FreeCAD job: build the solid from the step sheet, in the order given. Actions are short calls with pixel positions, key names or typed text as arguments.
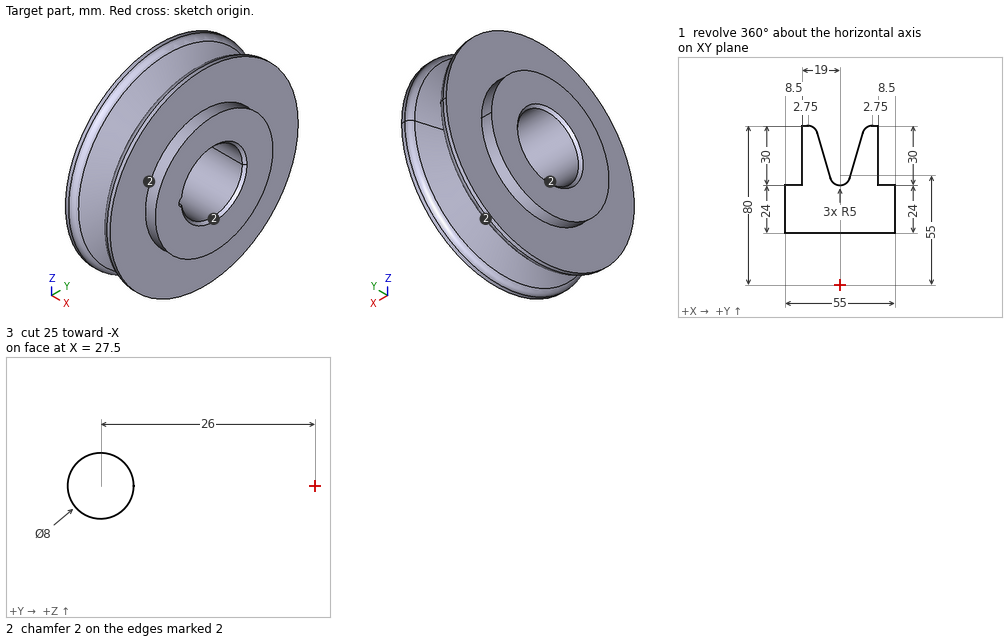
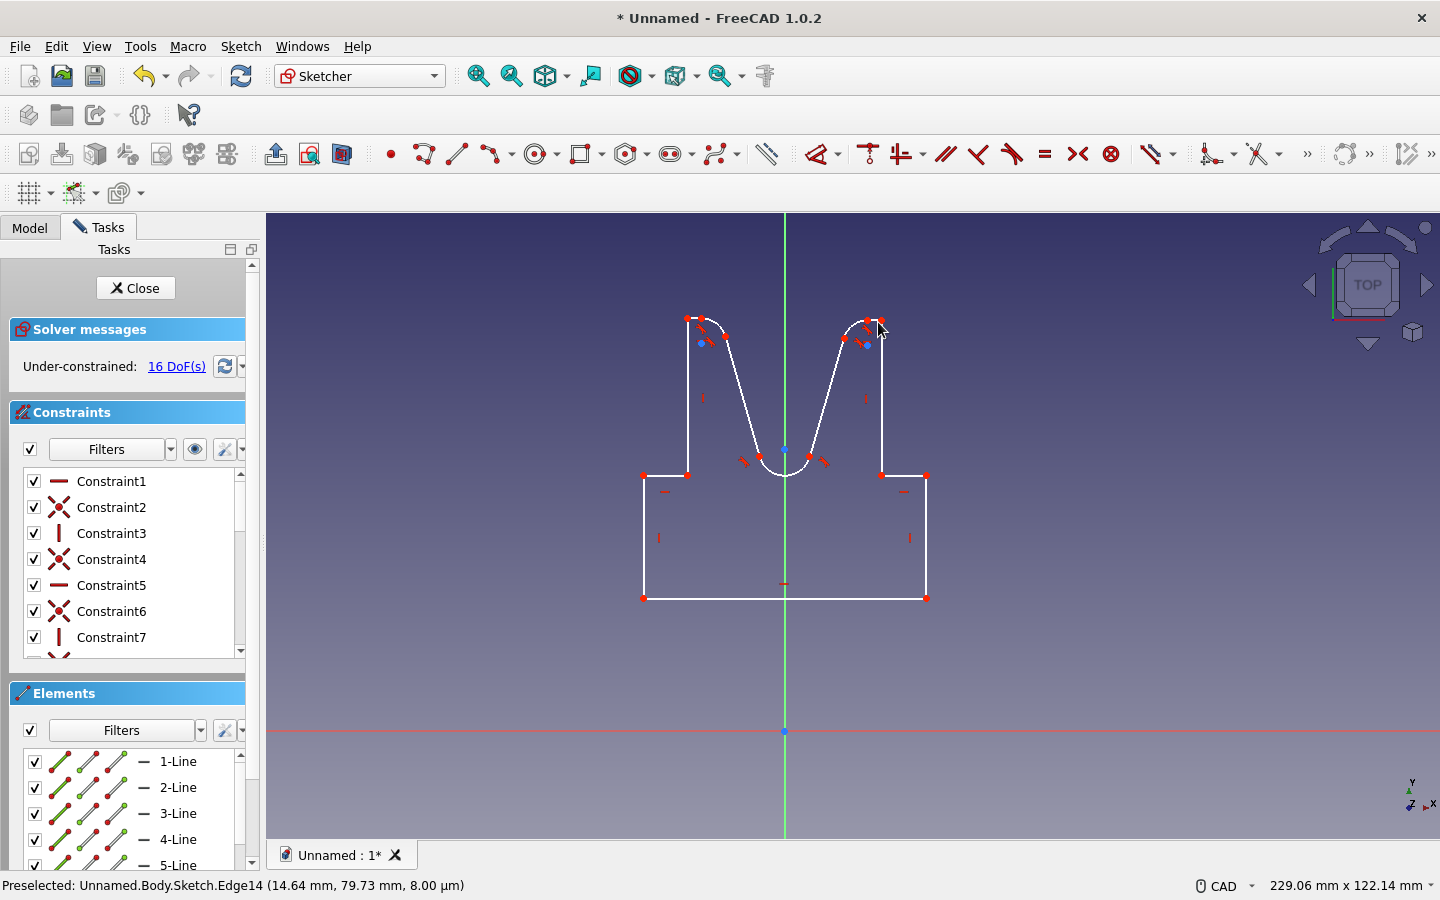
click(767, 468)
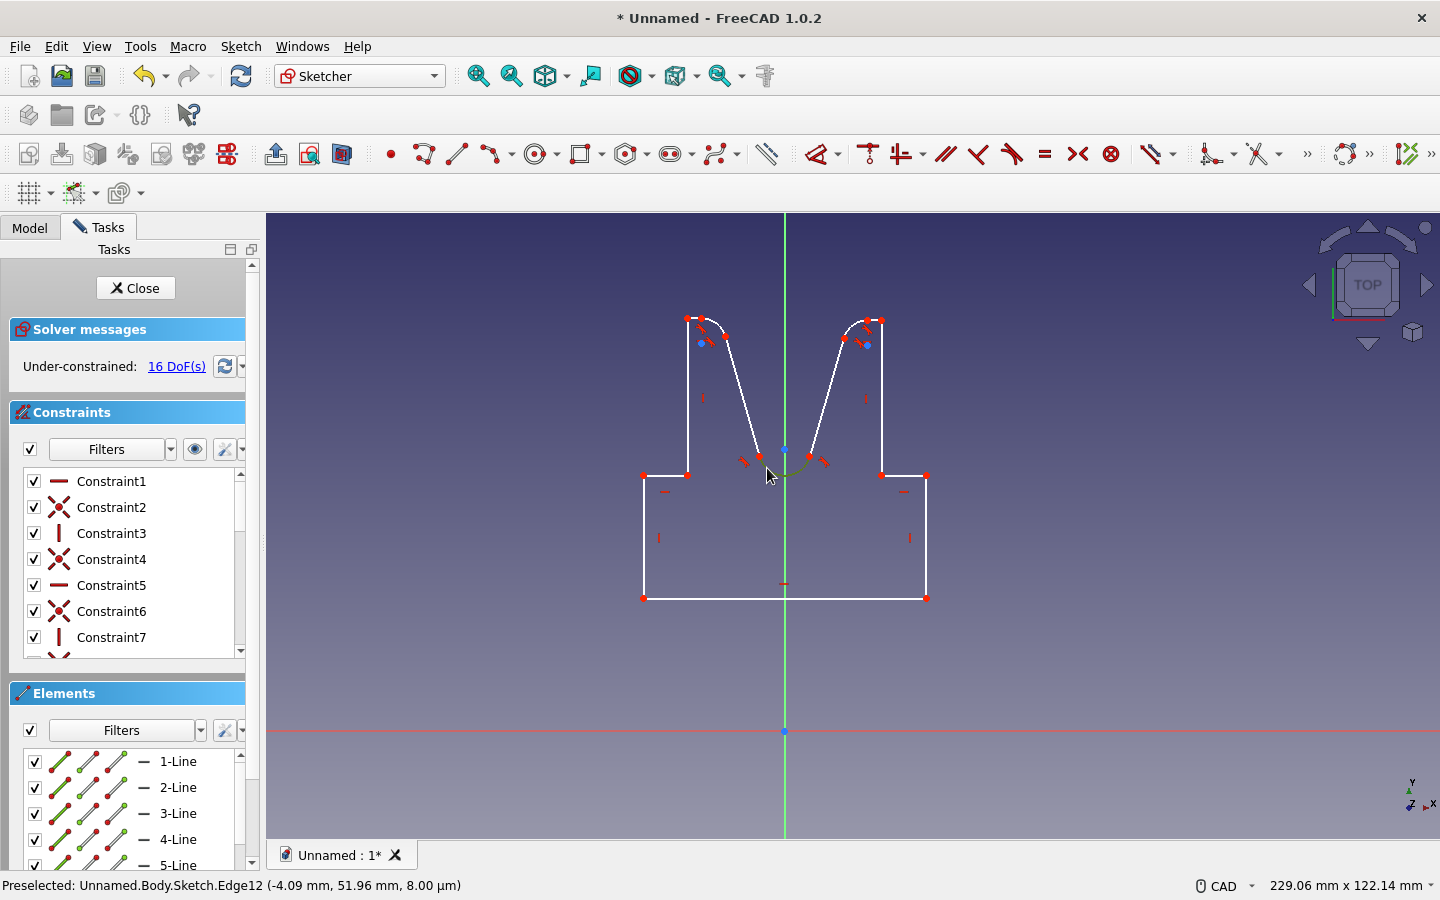
scroll(721, 328, up, 2)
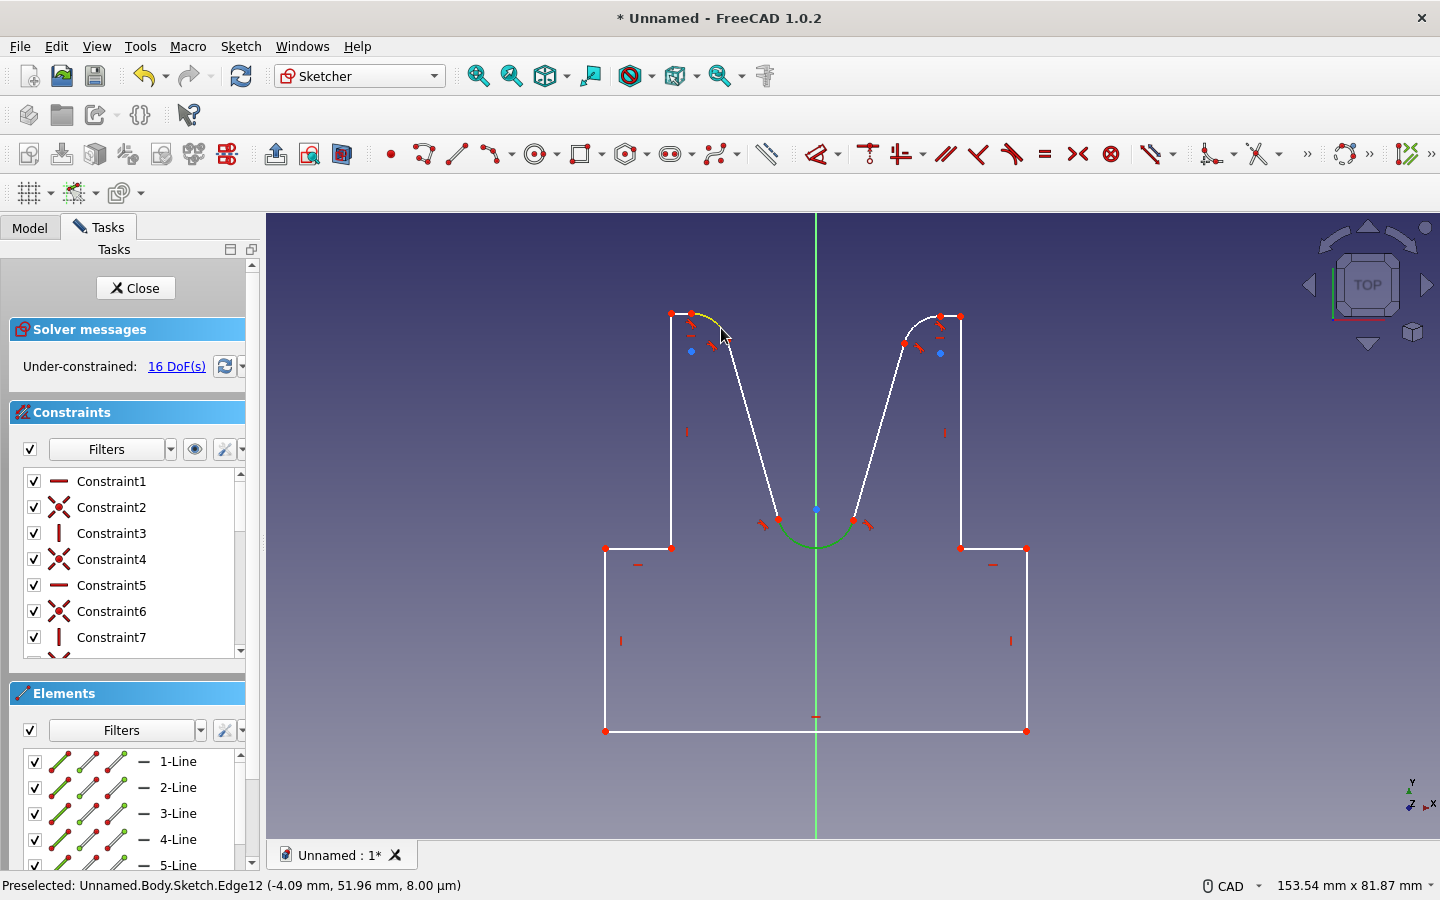
click(721, 328)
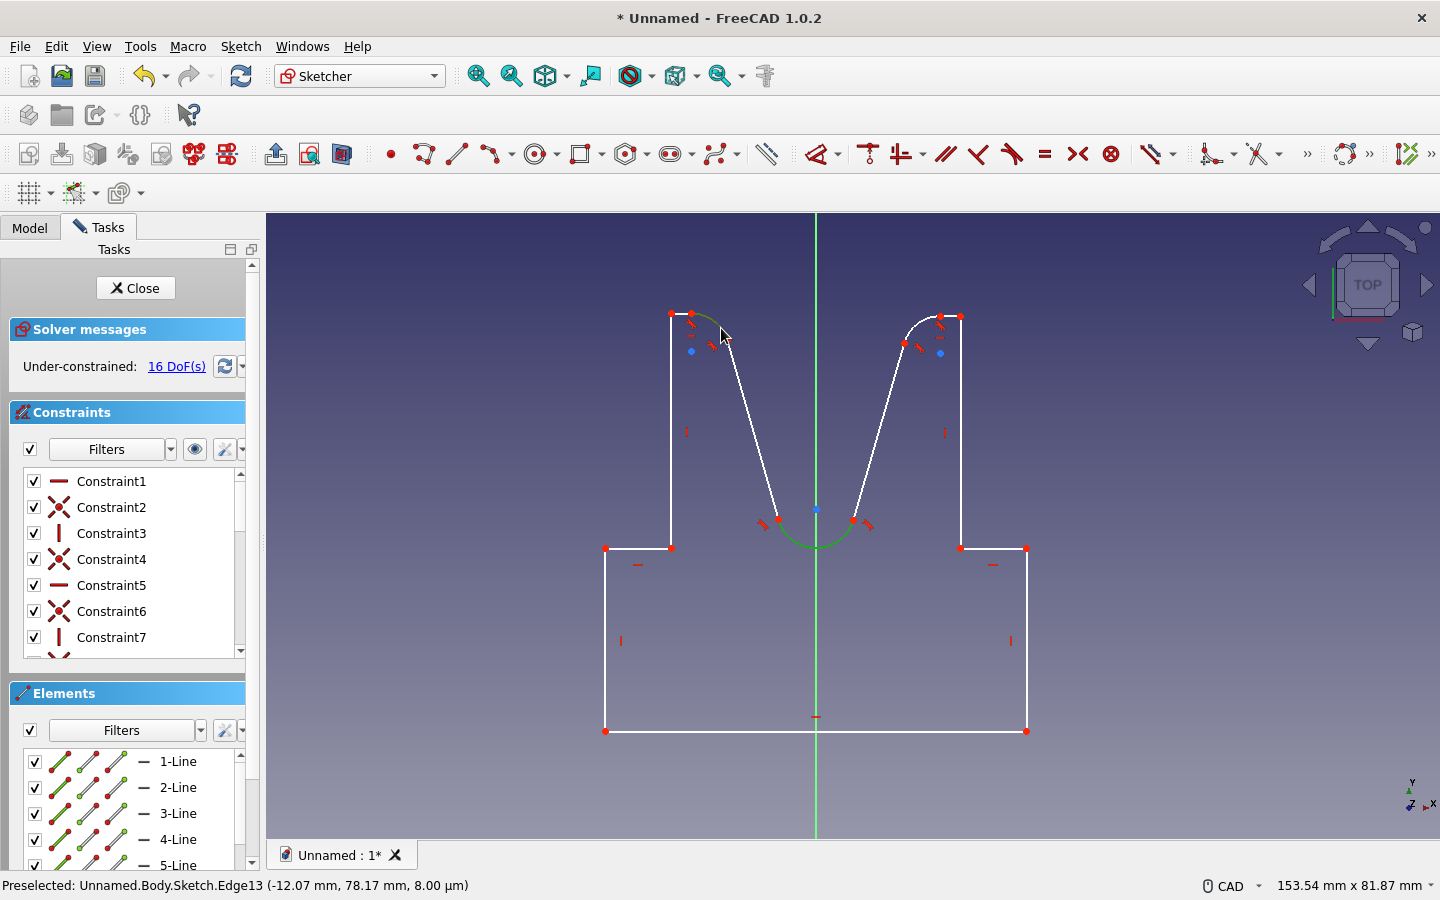
click(926, 319)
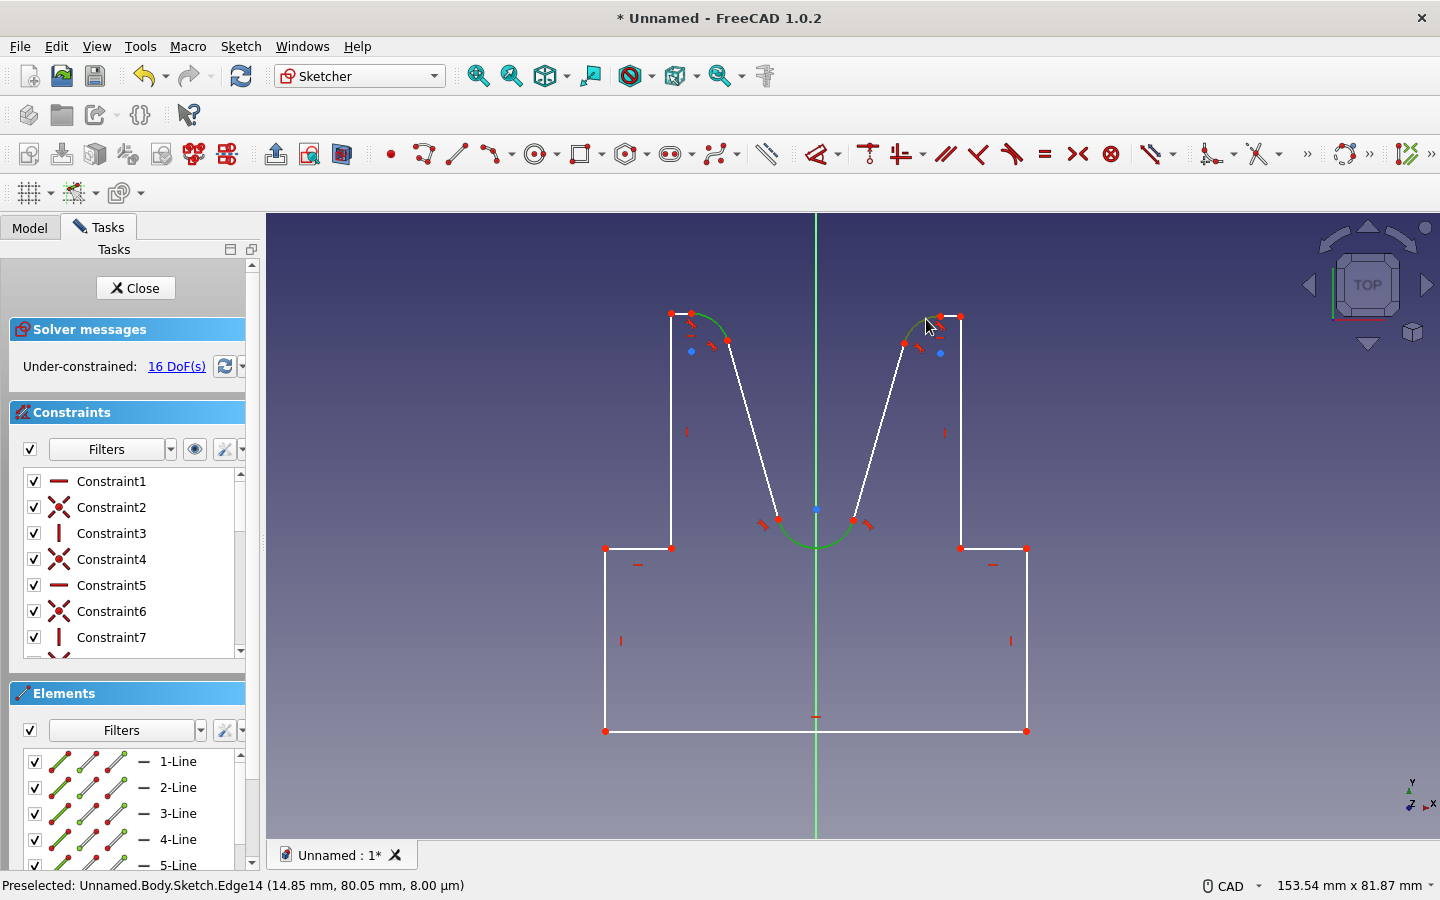
key(e)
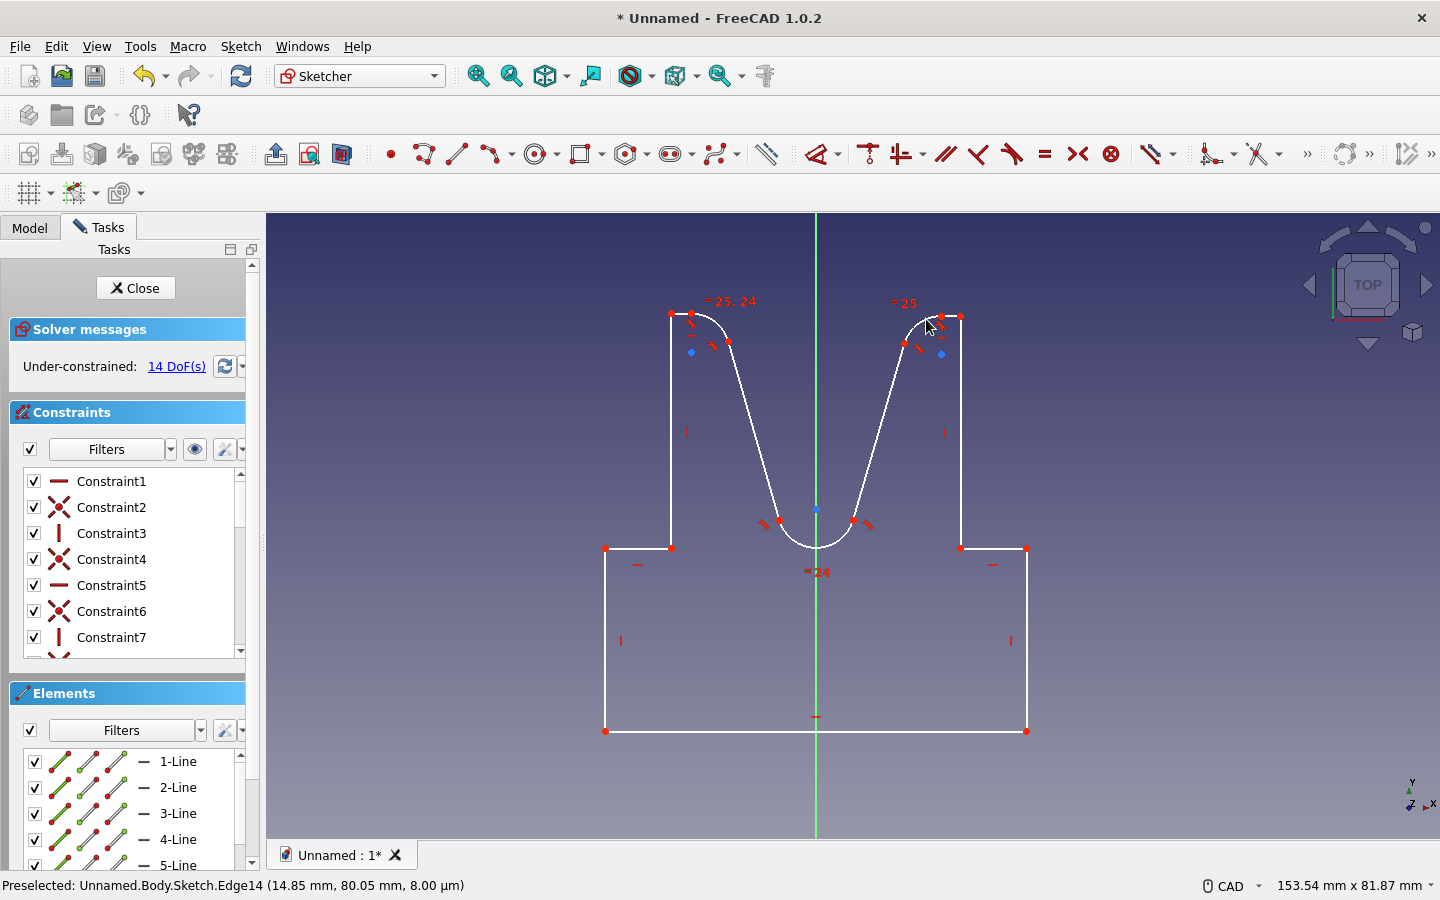
click(816, 509)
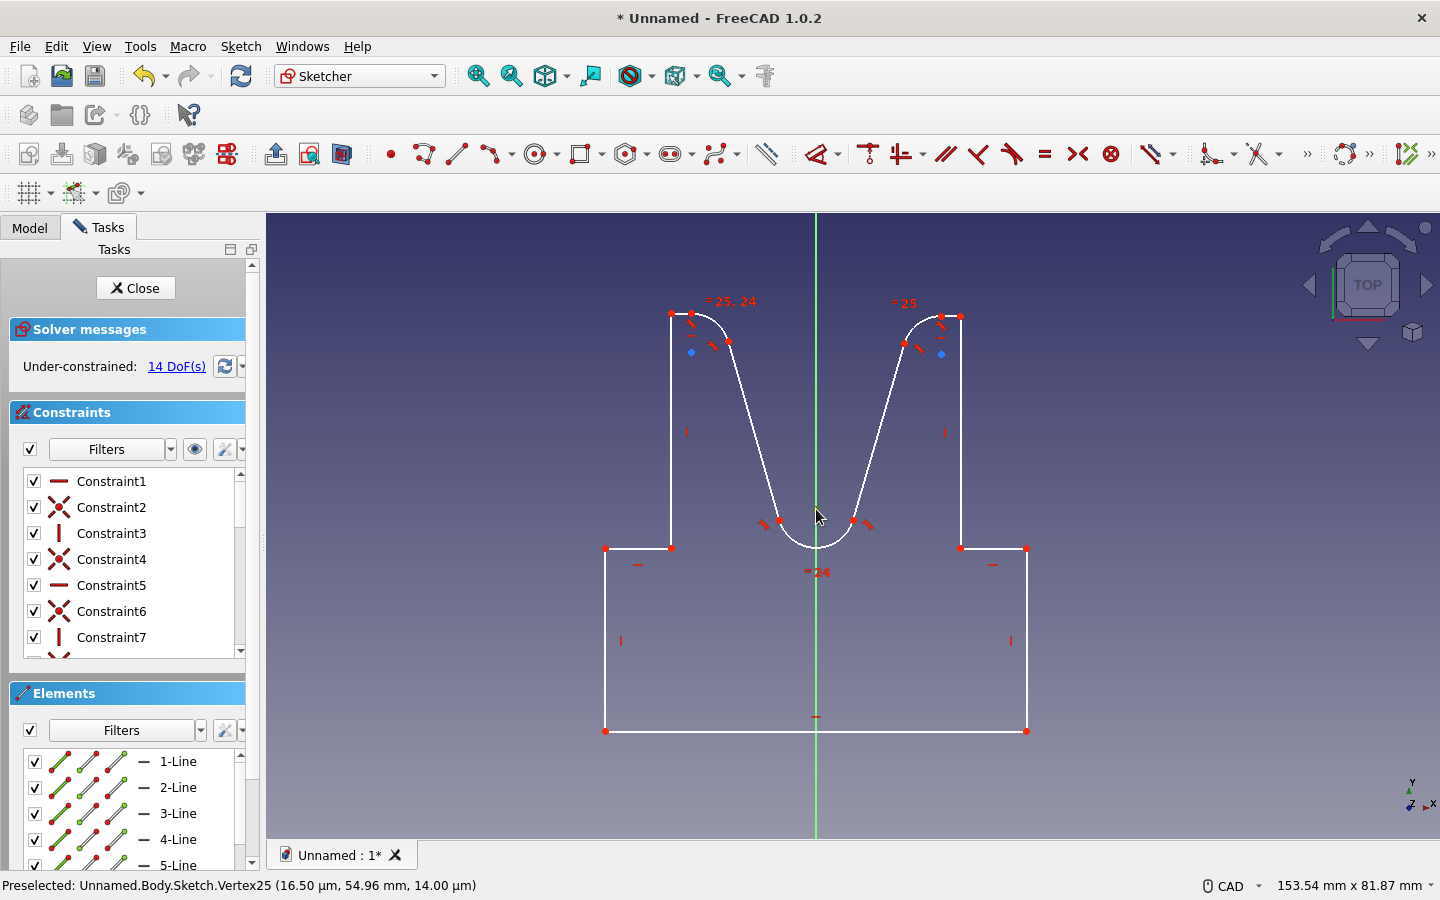
click(816, 770)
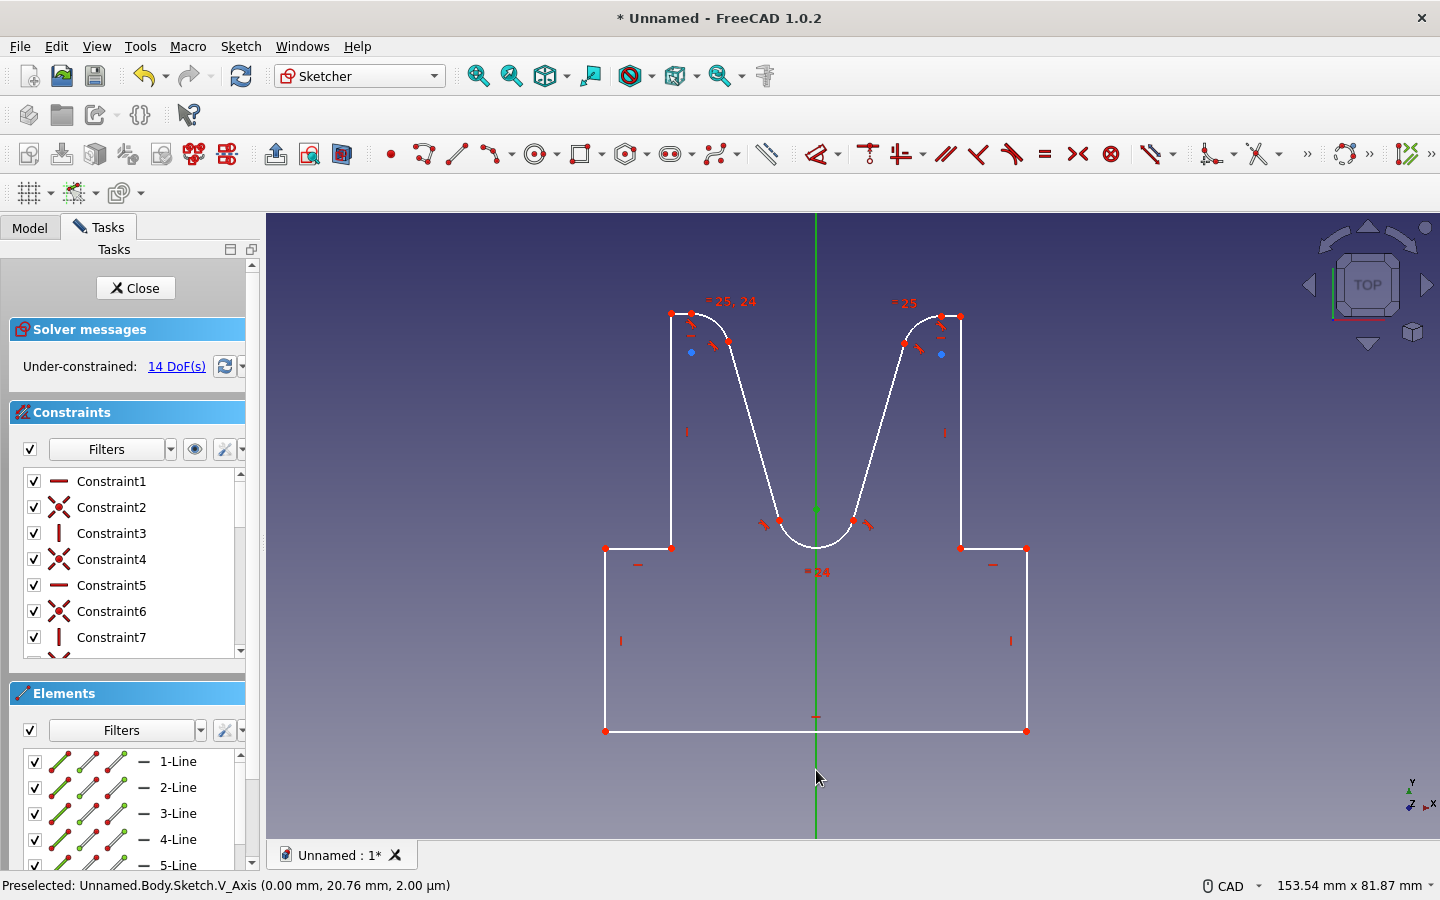
key(c)